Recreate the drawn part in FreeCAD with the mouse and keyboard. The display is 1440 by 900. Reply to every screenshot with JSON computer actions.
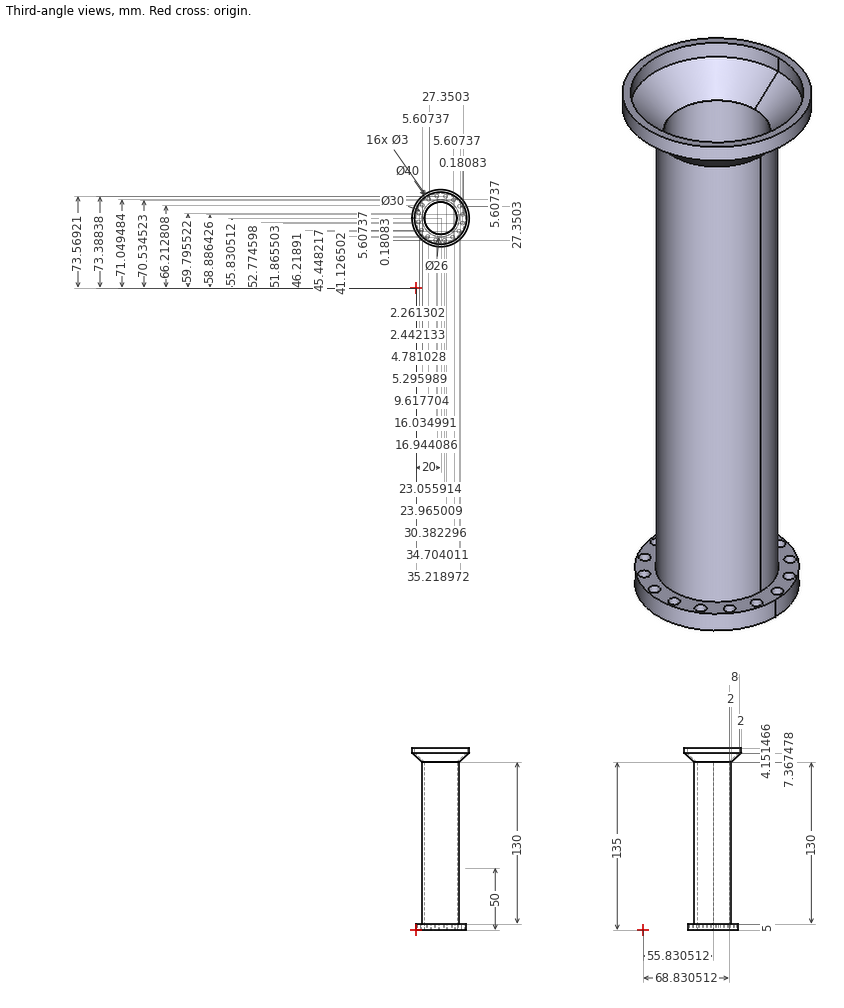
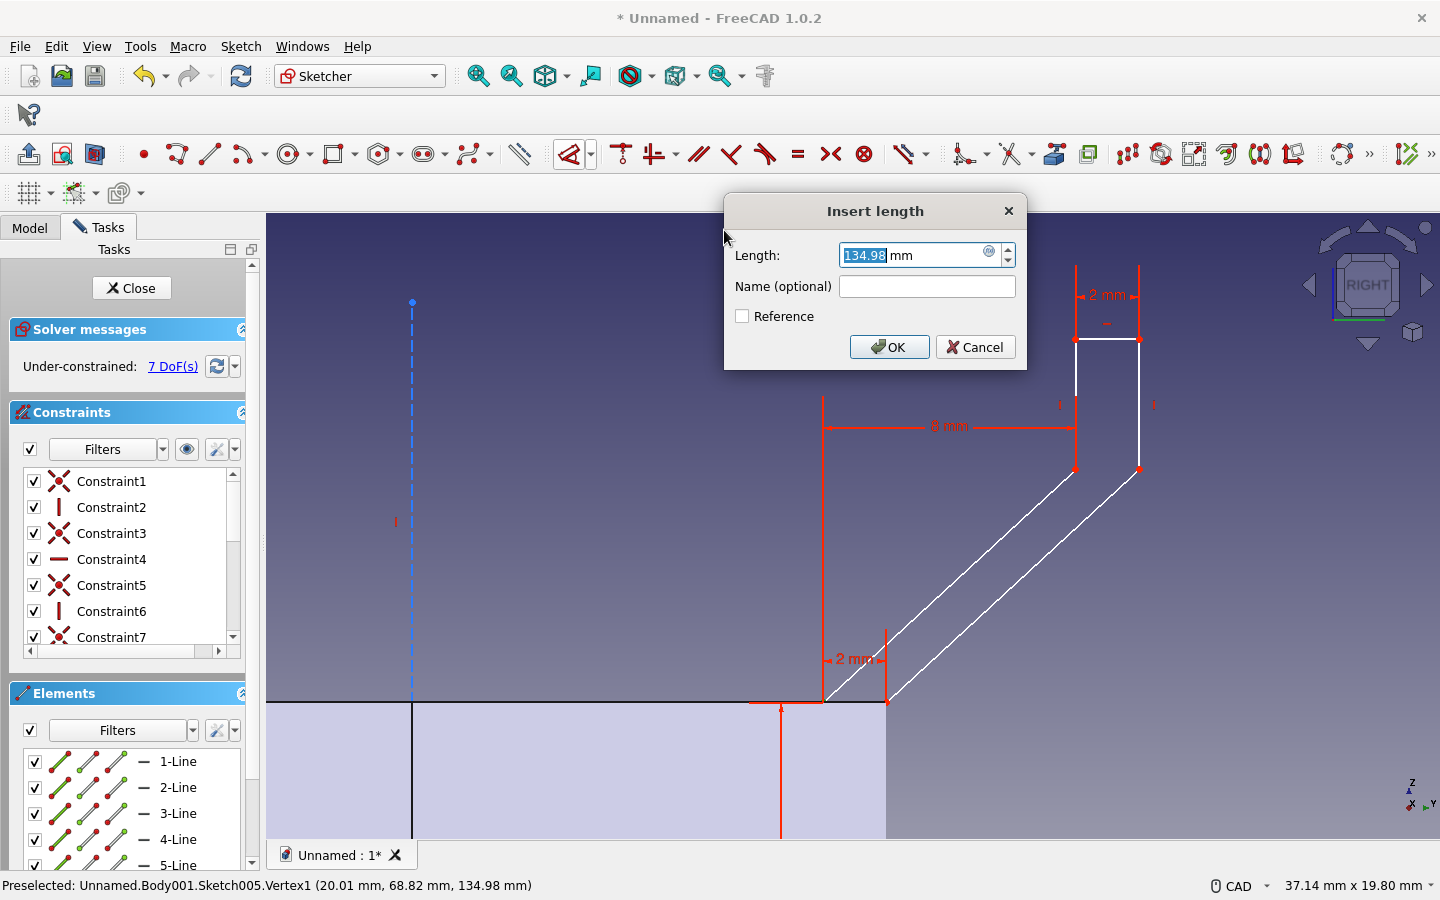
{"action": "type", "text": "135"}
{"action": "key", "text": "Return"}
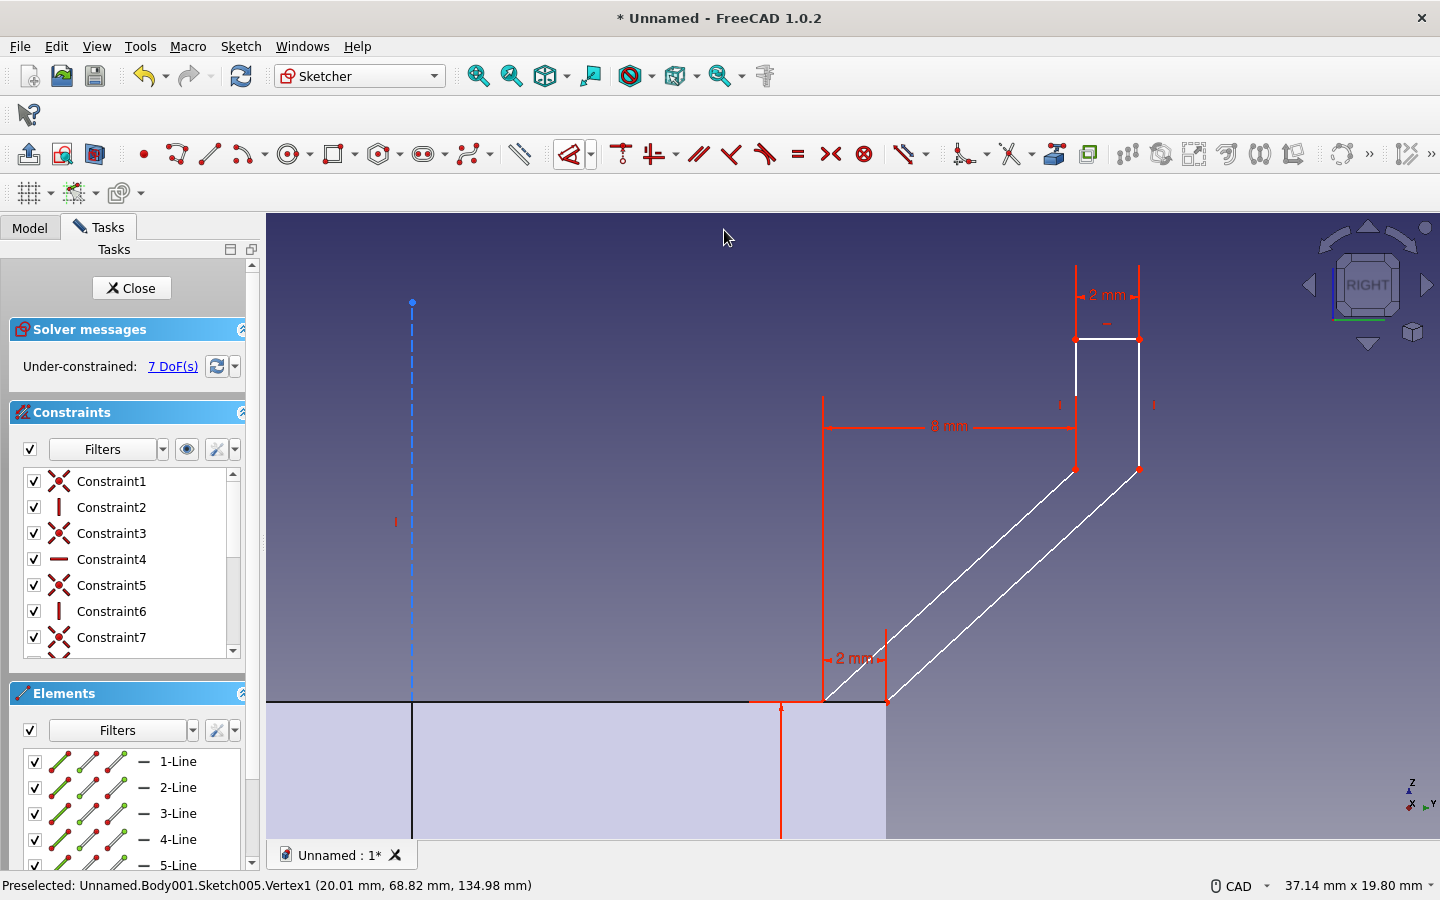
{"action": "left_click", "coordinate": [1076, 431]}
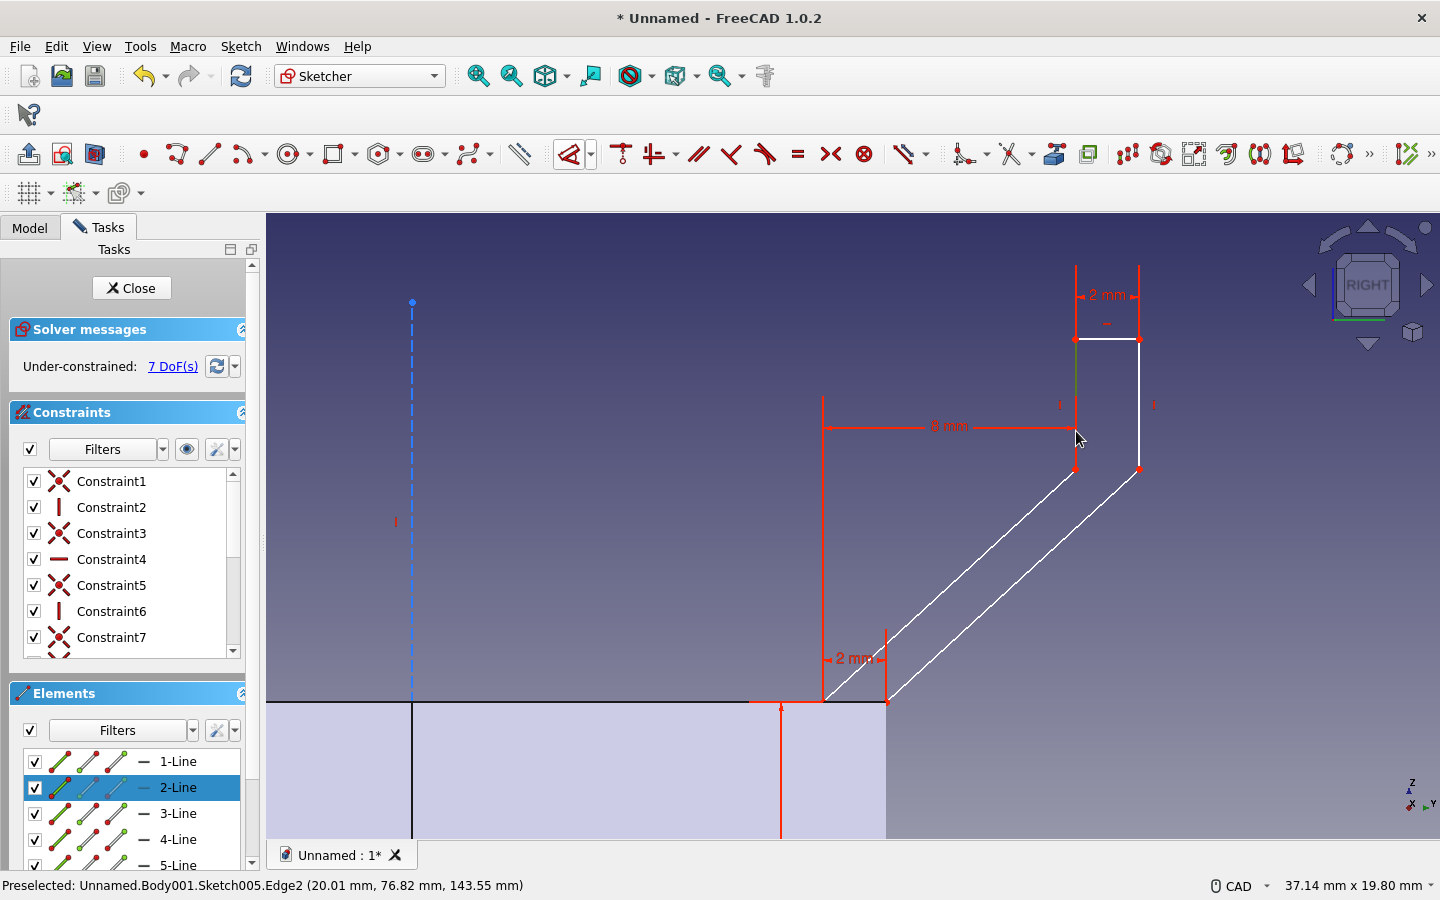
{"action": "key", "text": "i"}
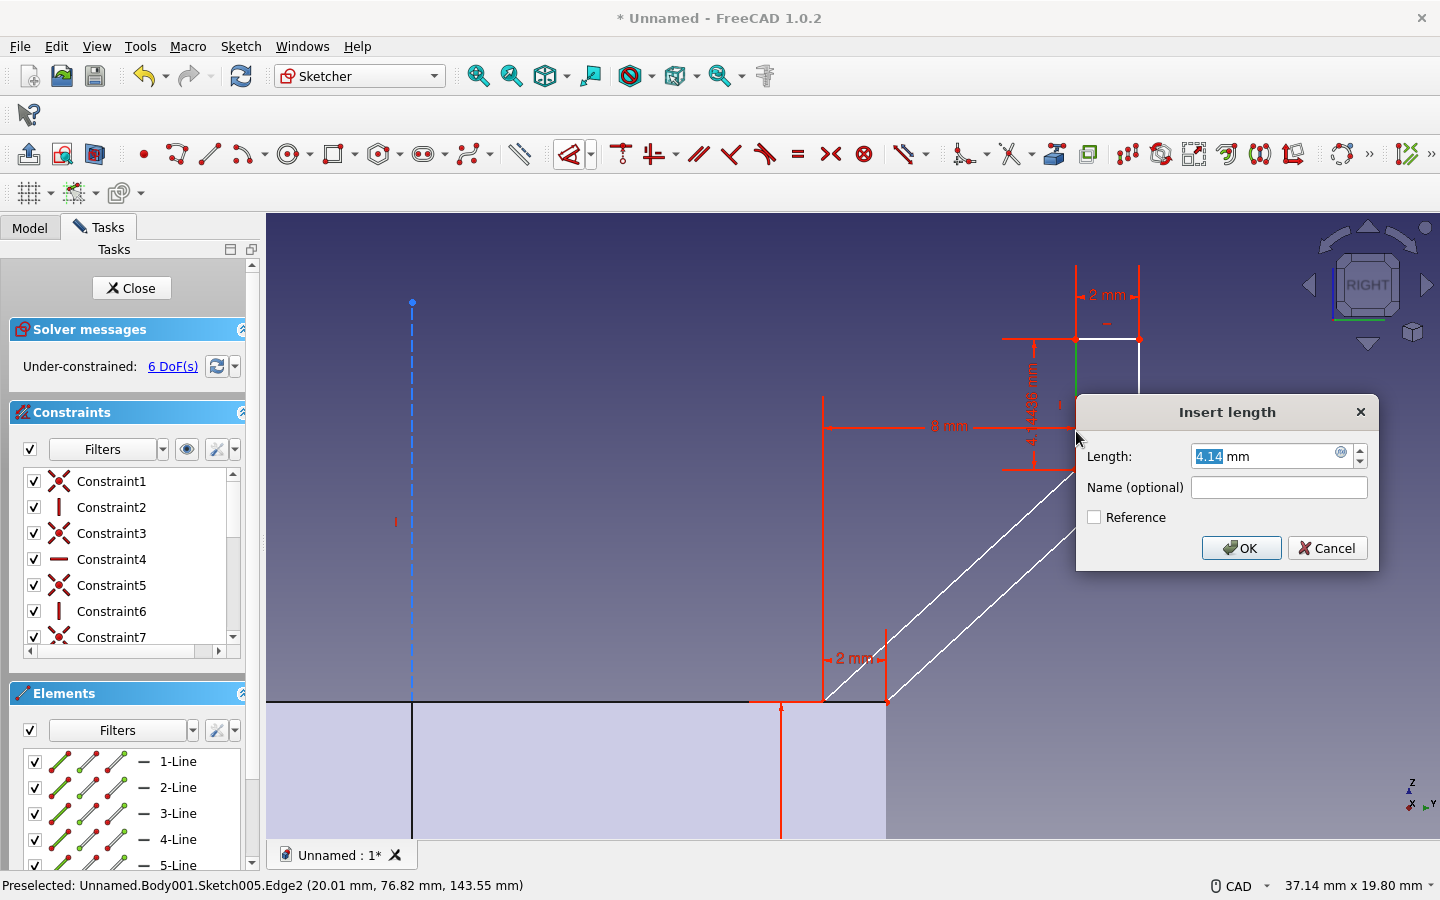
{"action": "type", "text": "4.151466"}
{"action": "key", "text": "Return"}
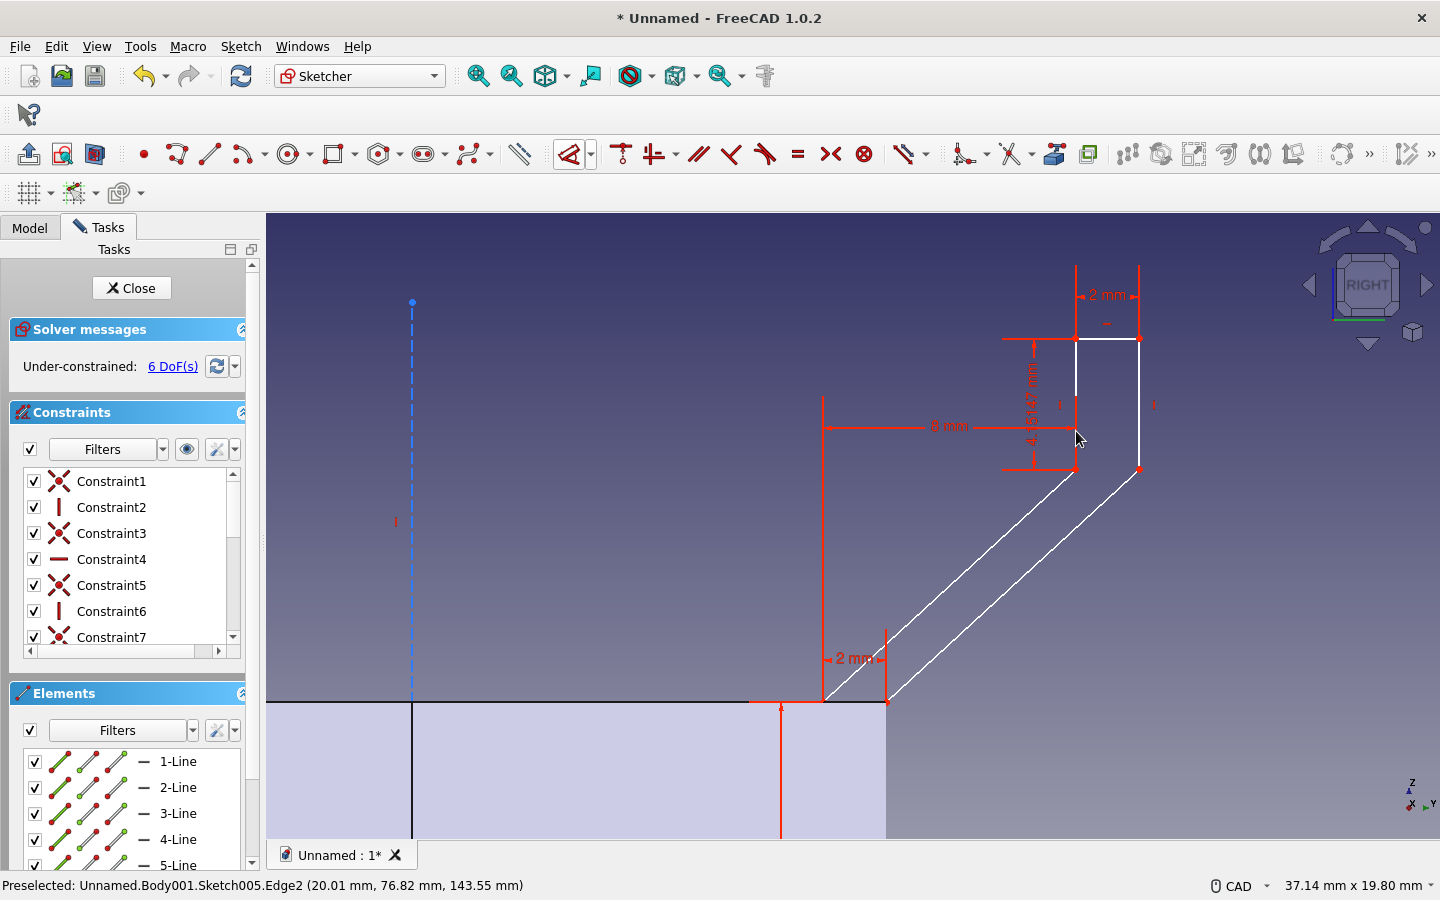
{"action": "left_click", "coordinate": [1139, 378]}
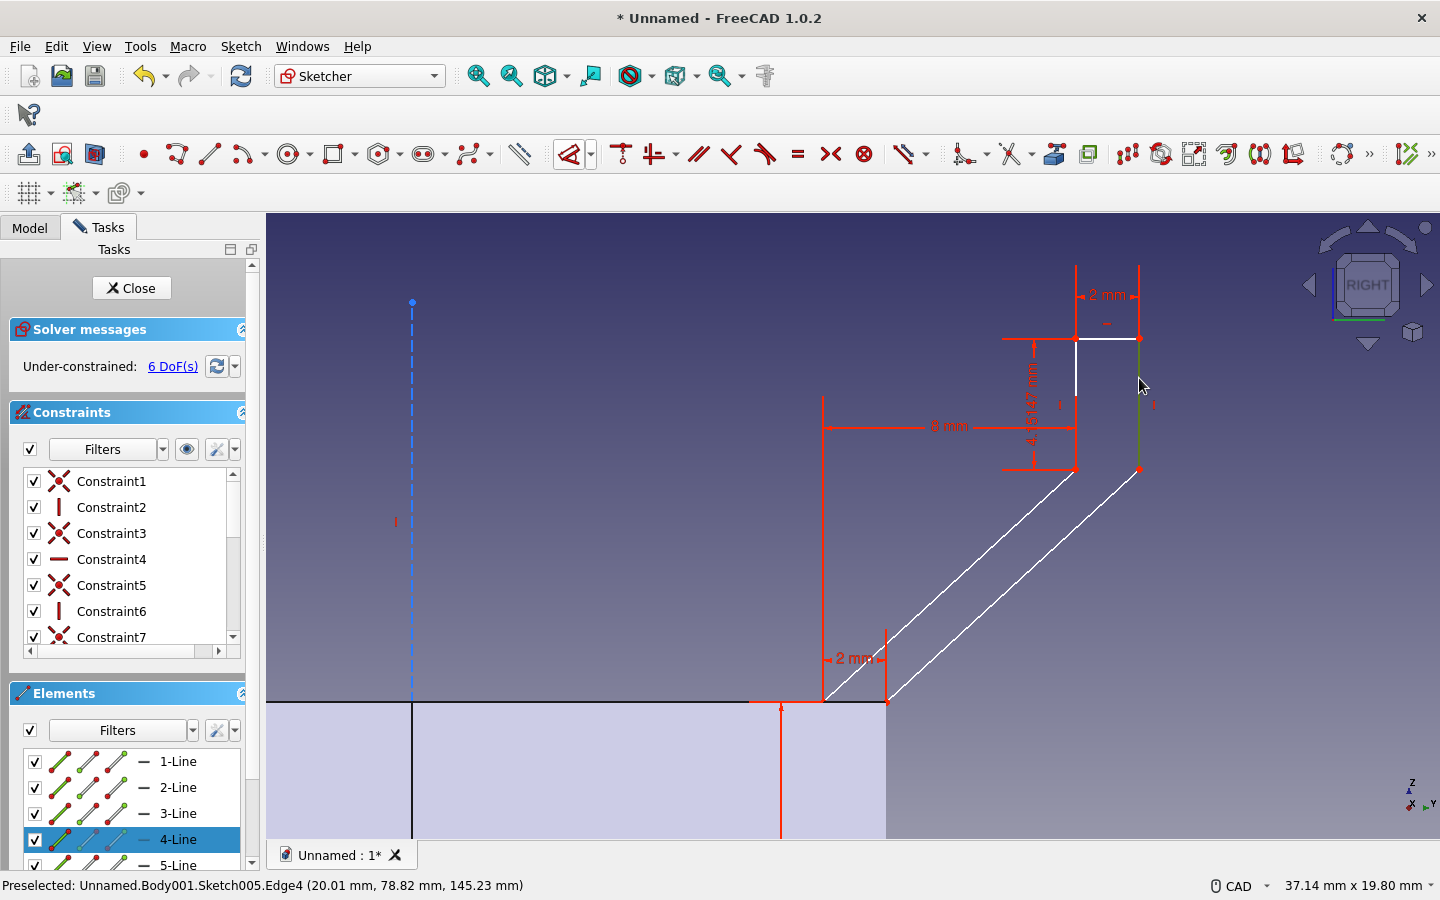
{"action": "left_click", "coordinate": [590, 154]}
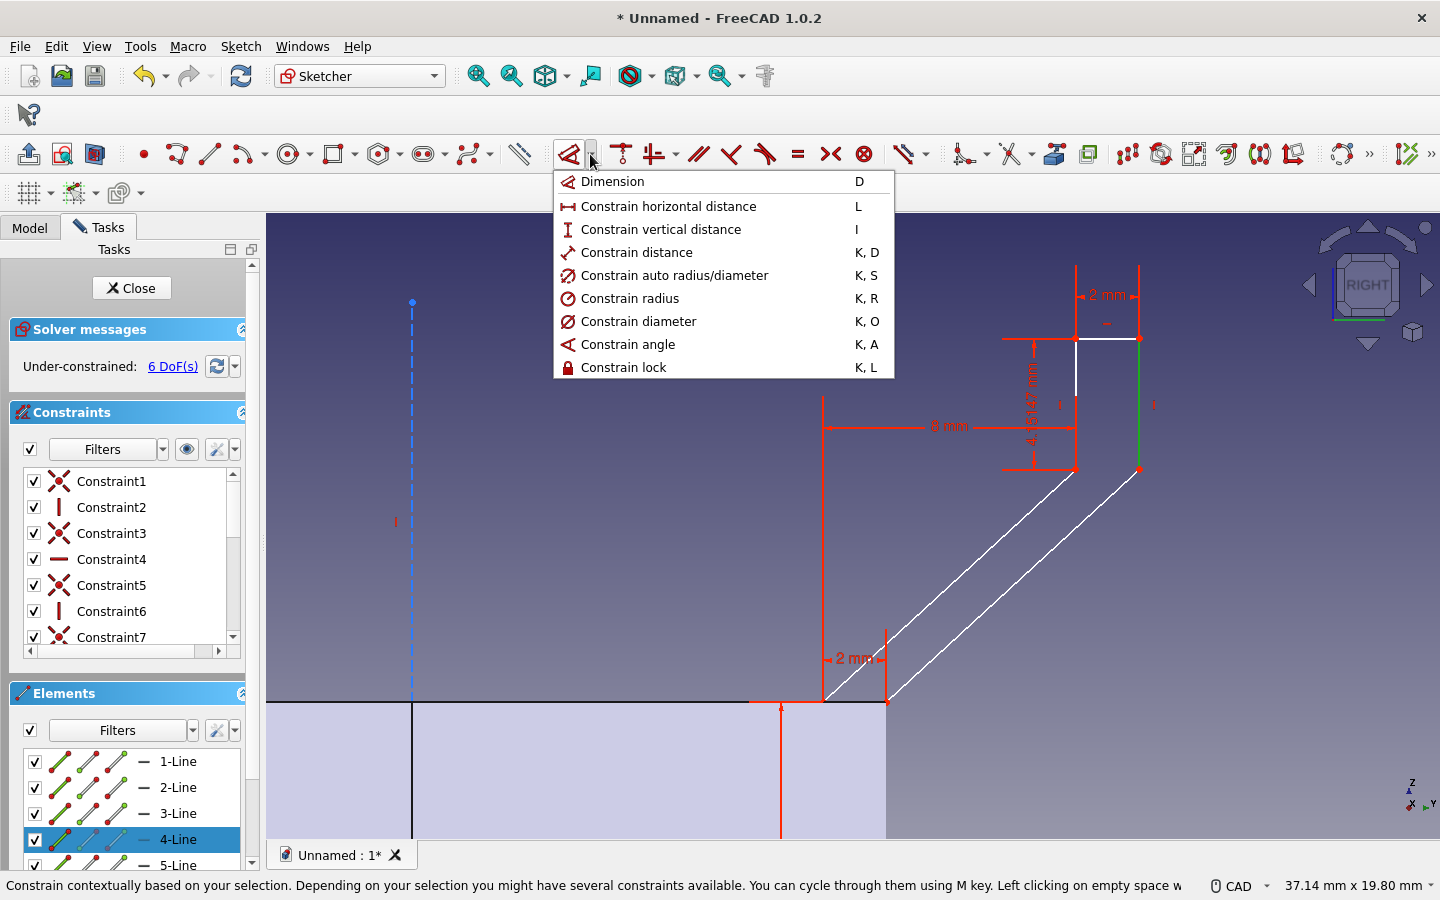
{"action": "left_click", "coordinate": [724, 230]}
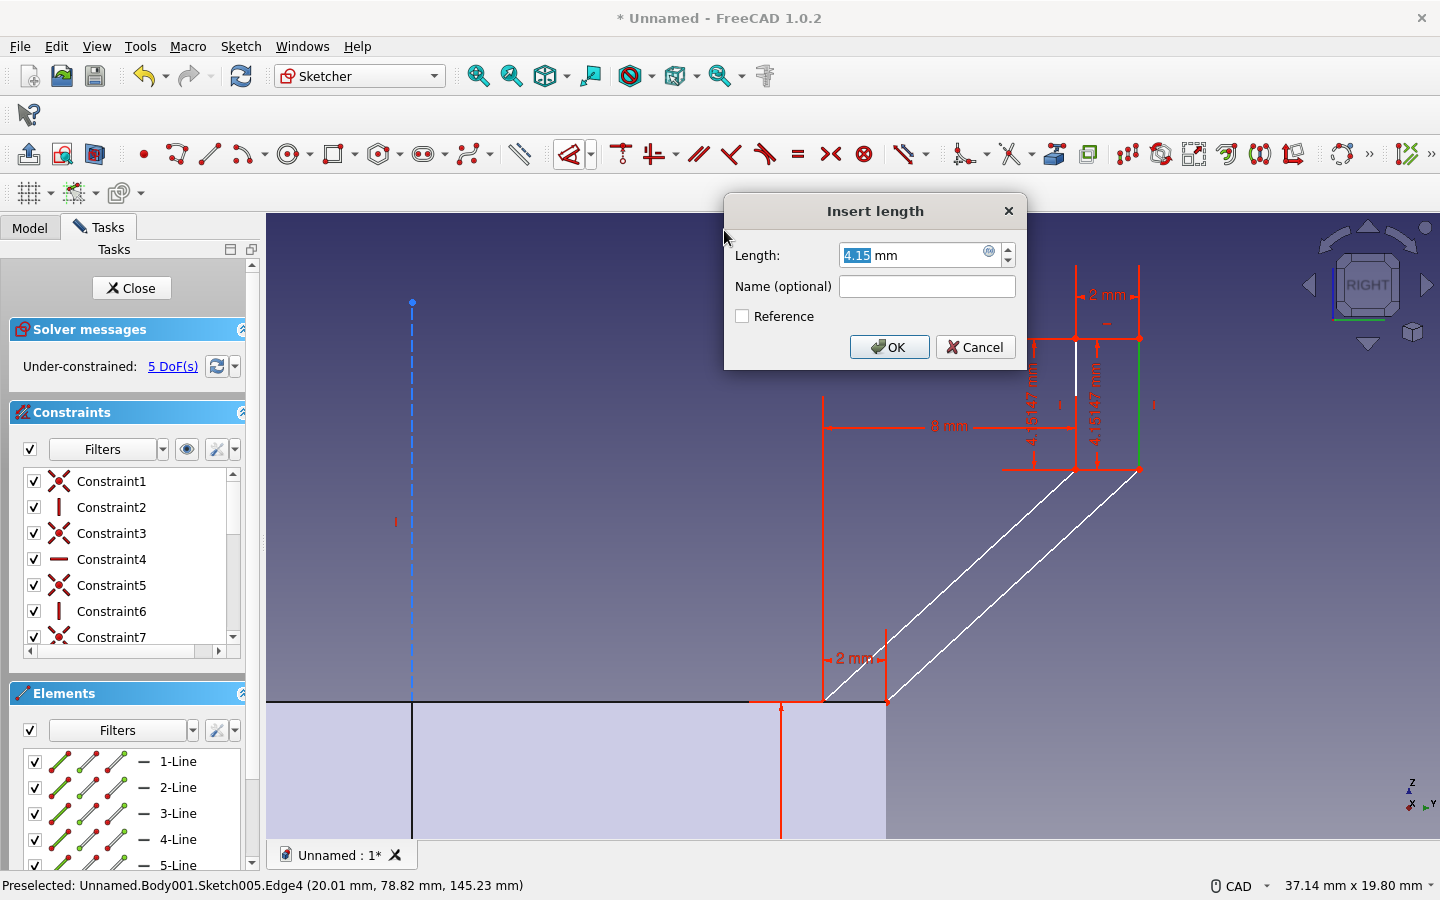
{"action": "type", "text": "4.151466"}
{"action": "key", "text": "Return"}